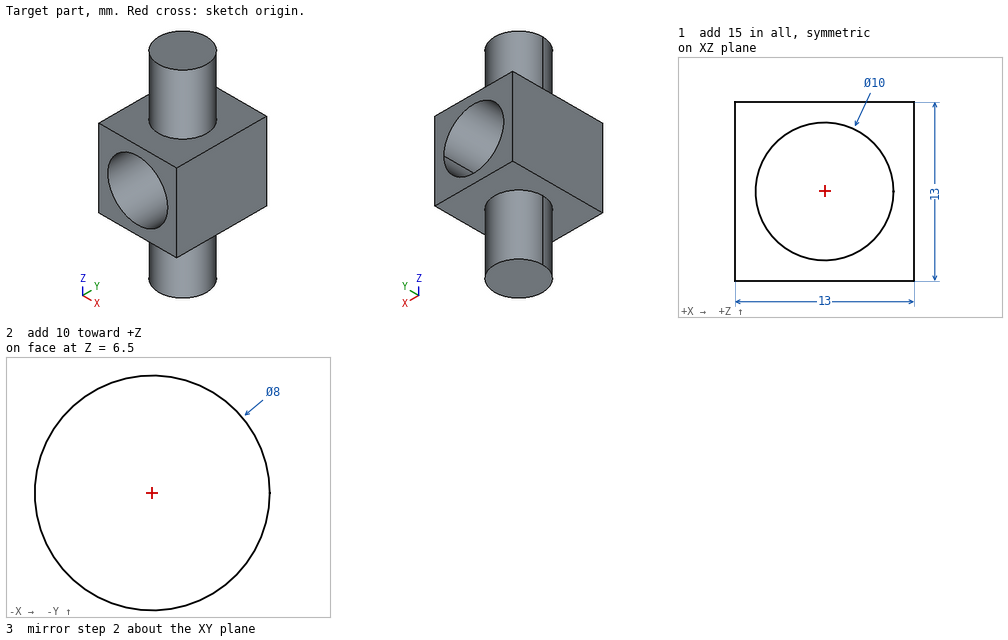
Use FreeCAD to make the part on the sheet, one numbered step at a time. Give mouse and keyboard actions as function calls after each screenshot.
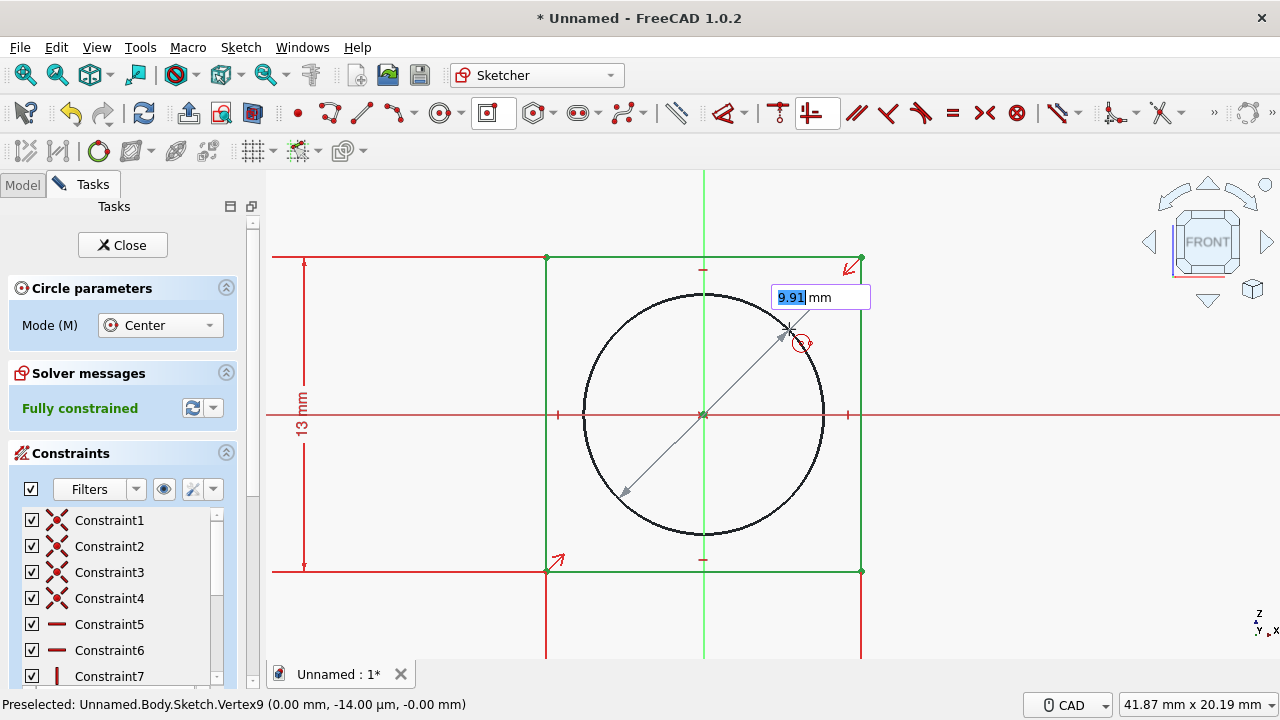
text(10)
key(Return)
key(Escape)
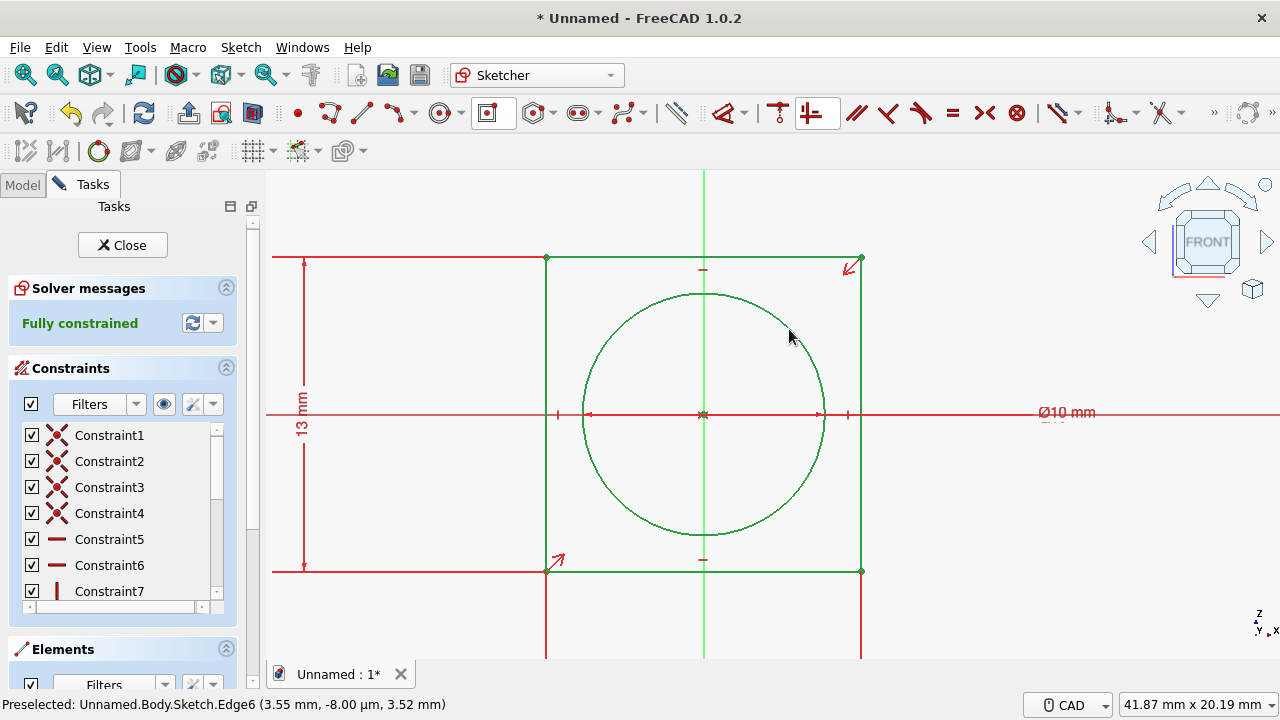
click(123, 245)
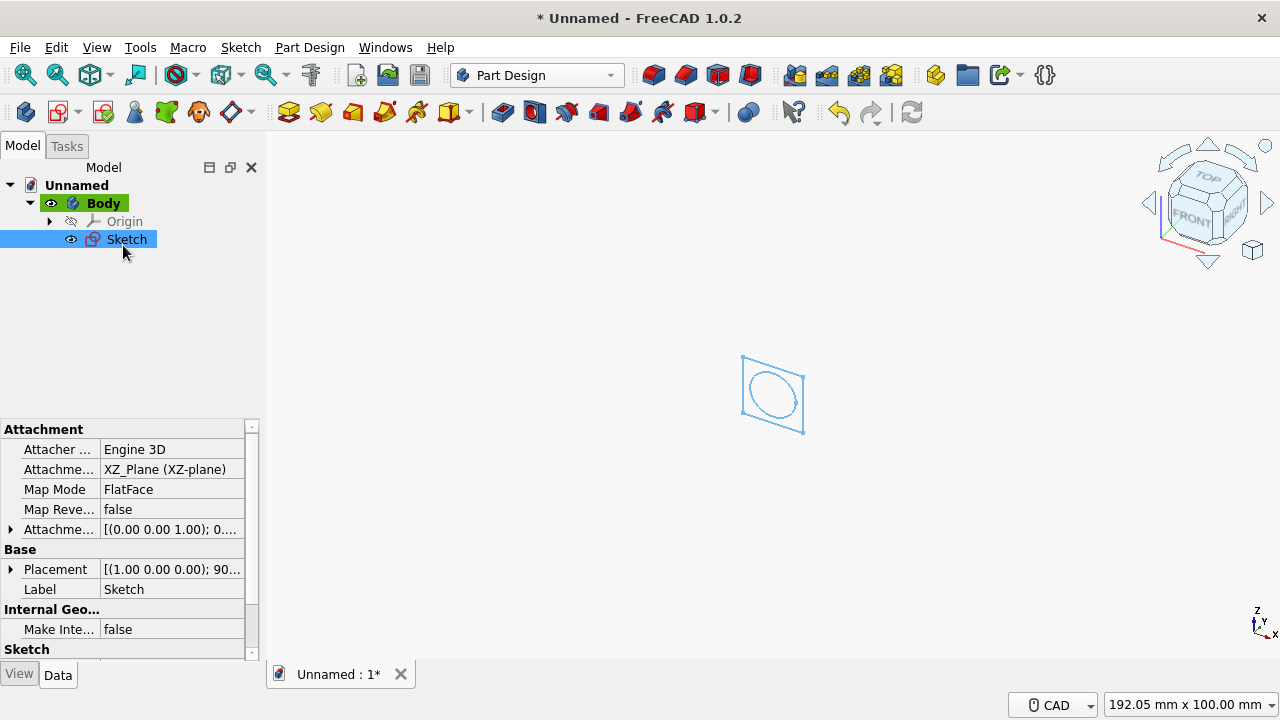
click(290, 112)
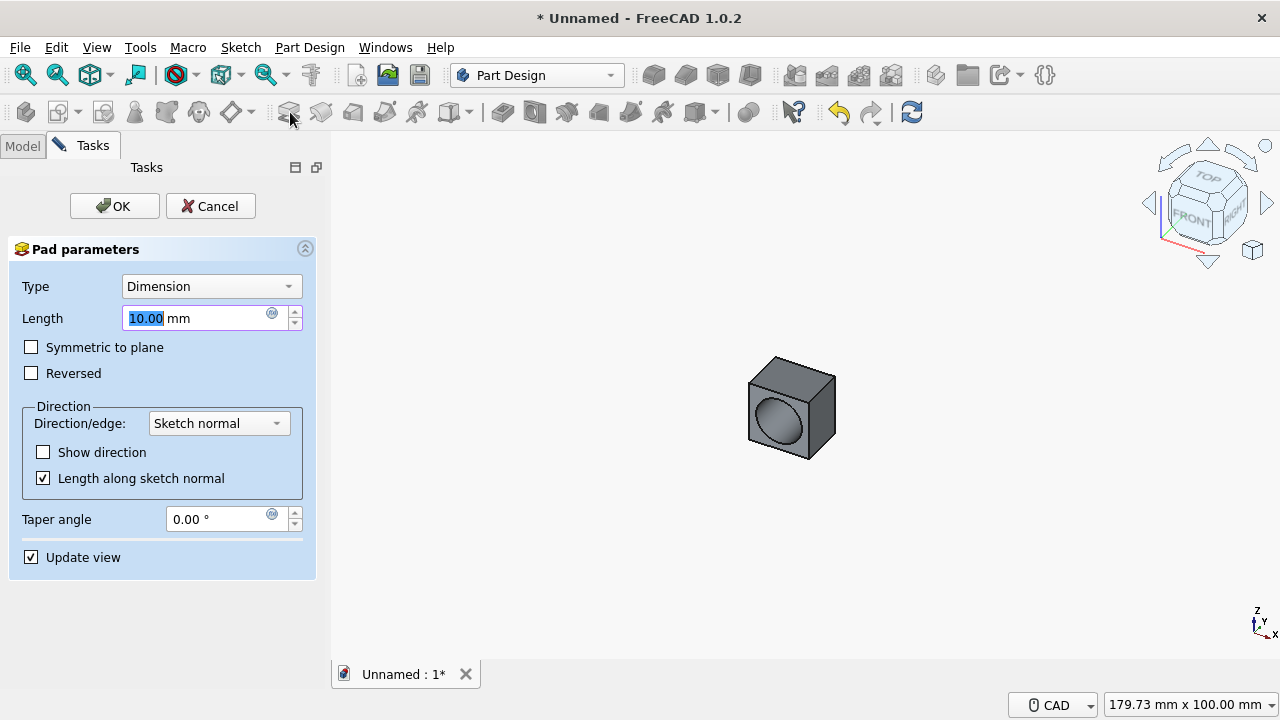
text(15)
key(Tab)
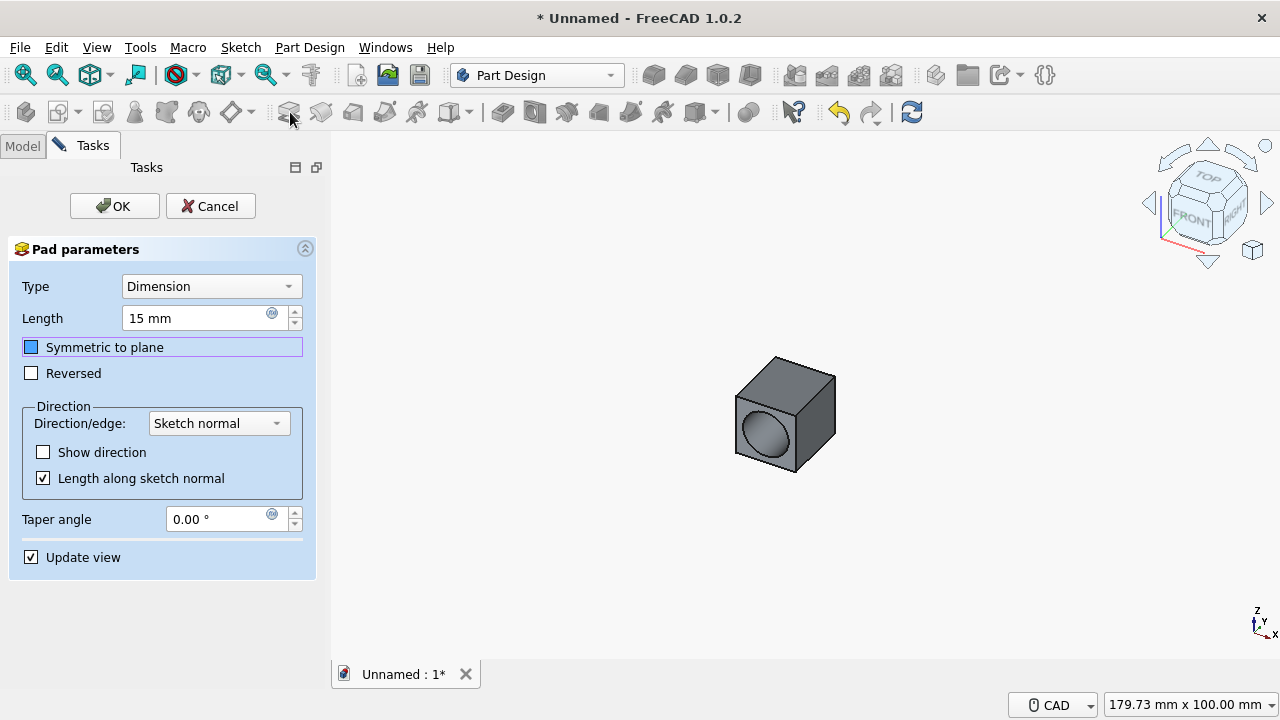
click(30, 347)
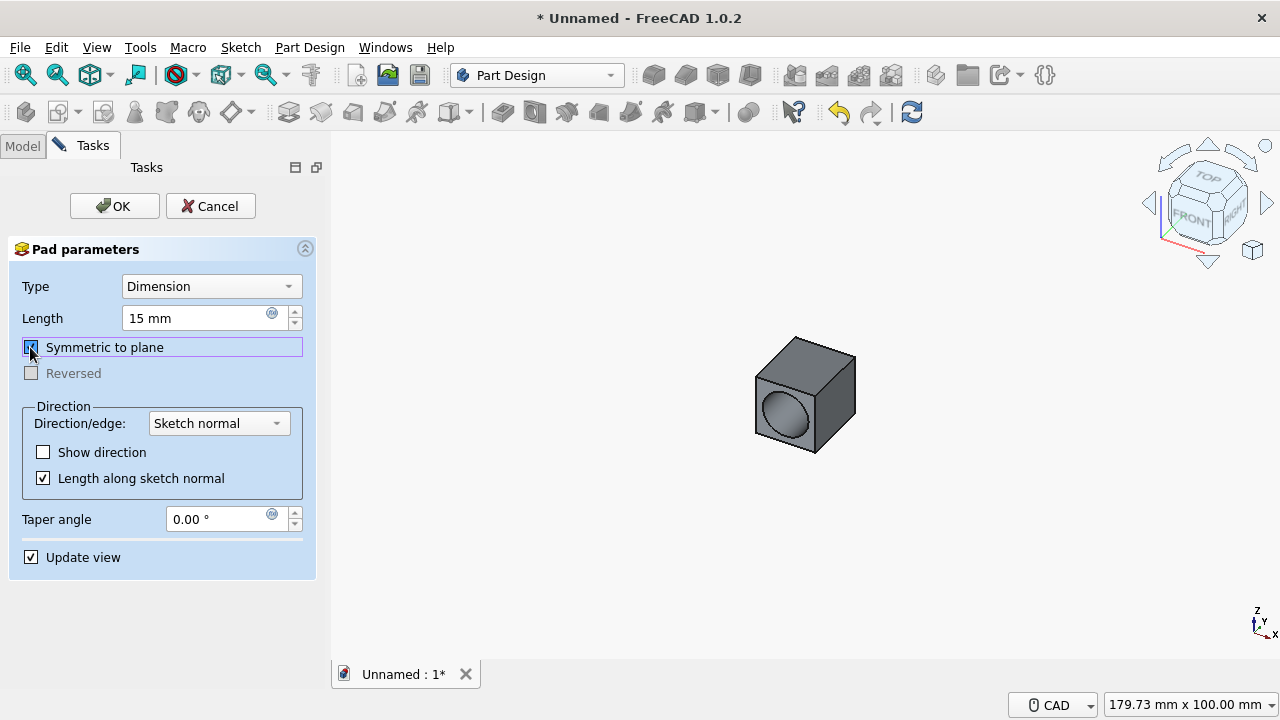
click(115, 206)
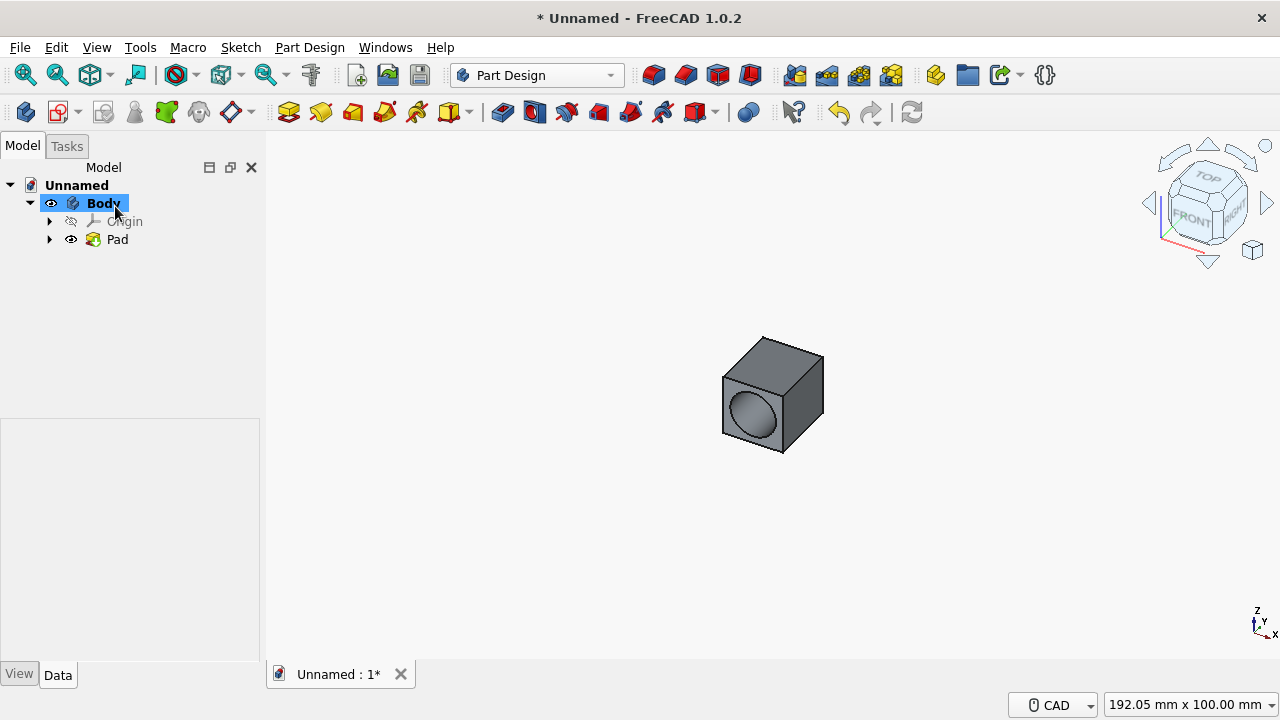
click(26, 76)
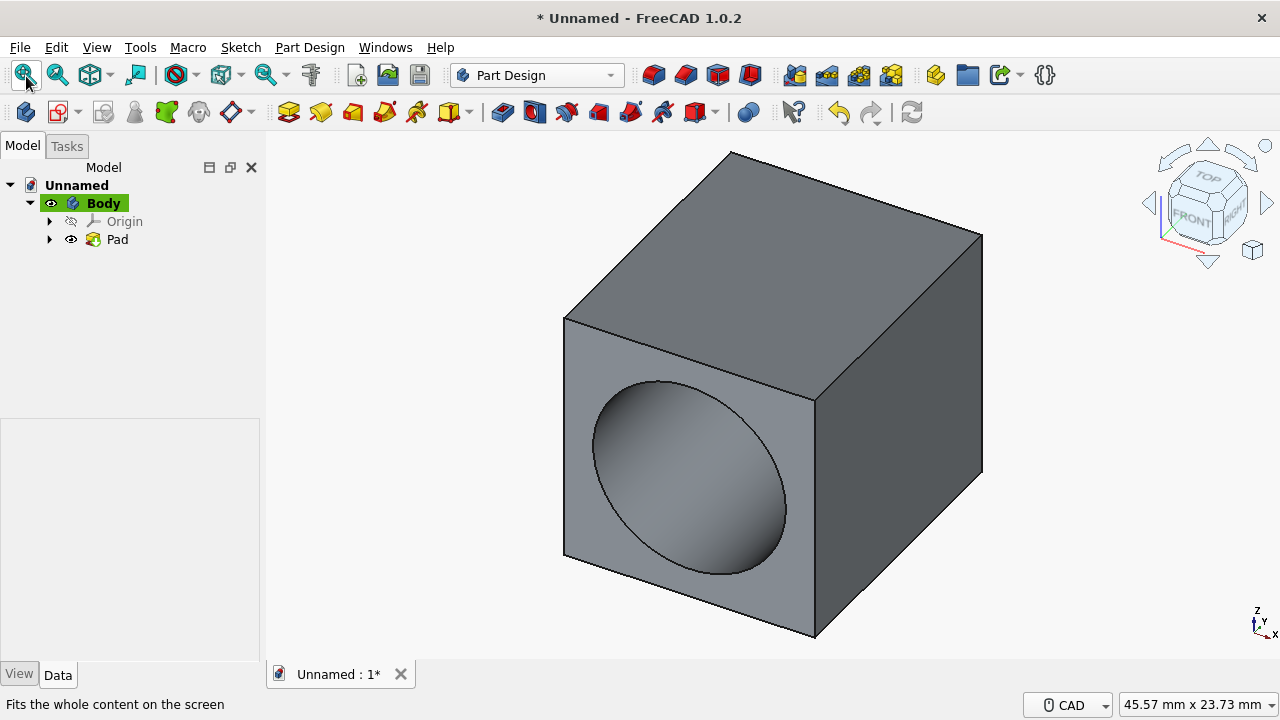
click(773, 276)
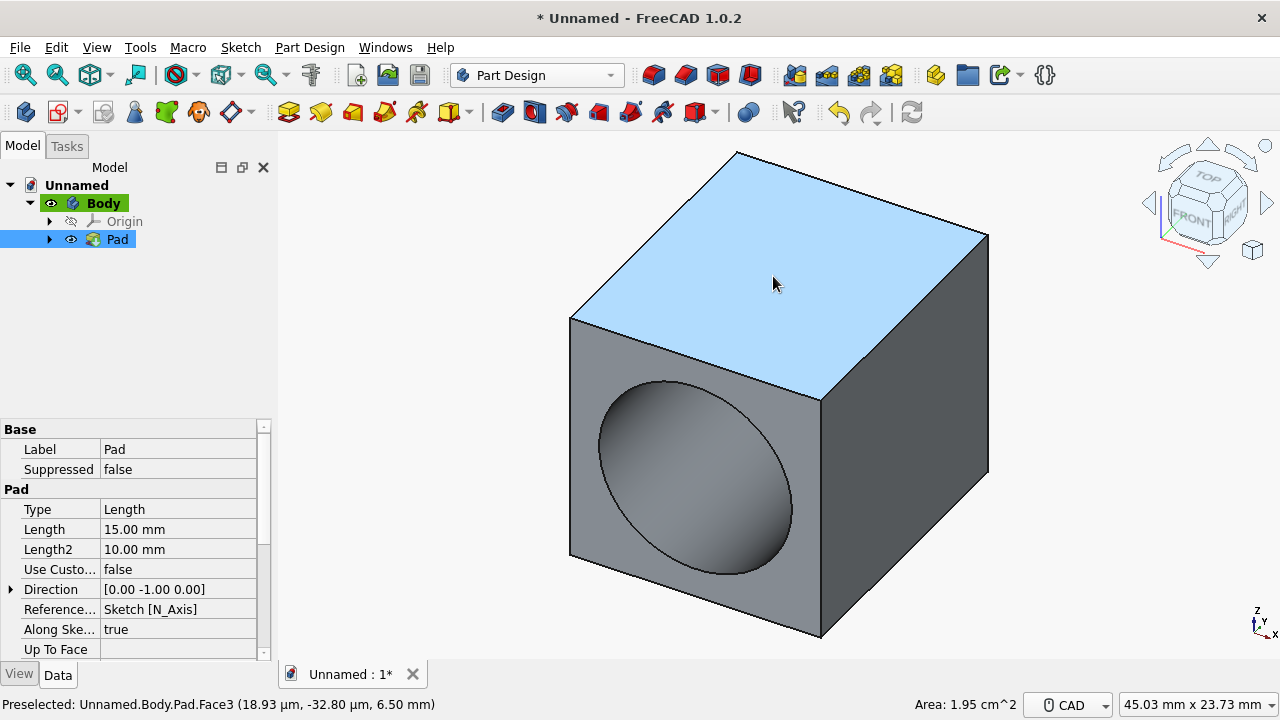
click(58, 112)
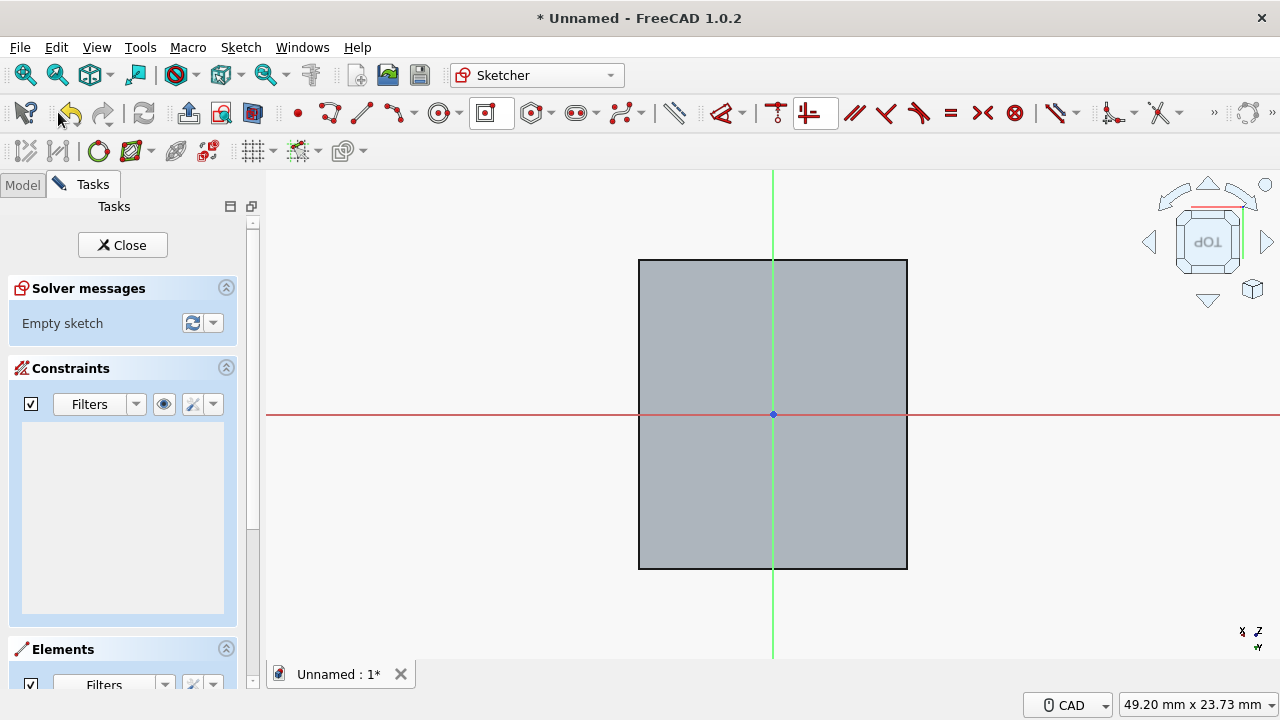
scroll(856, 415, up, 3)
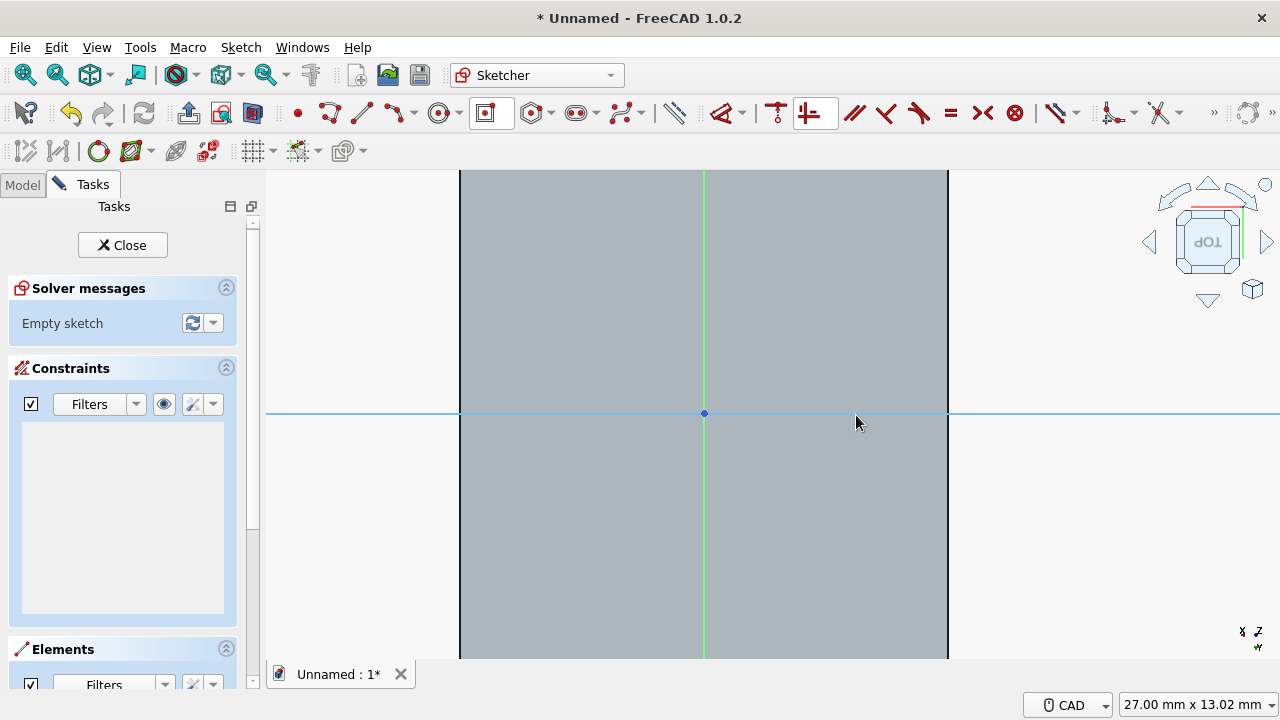
click(440, 114)